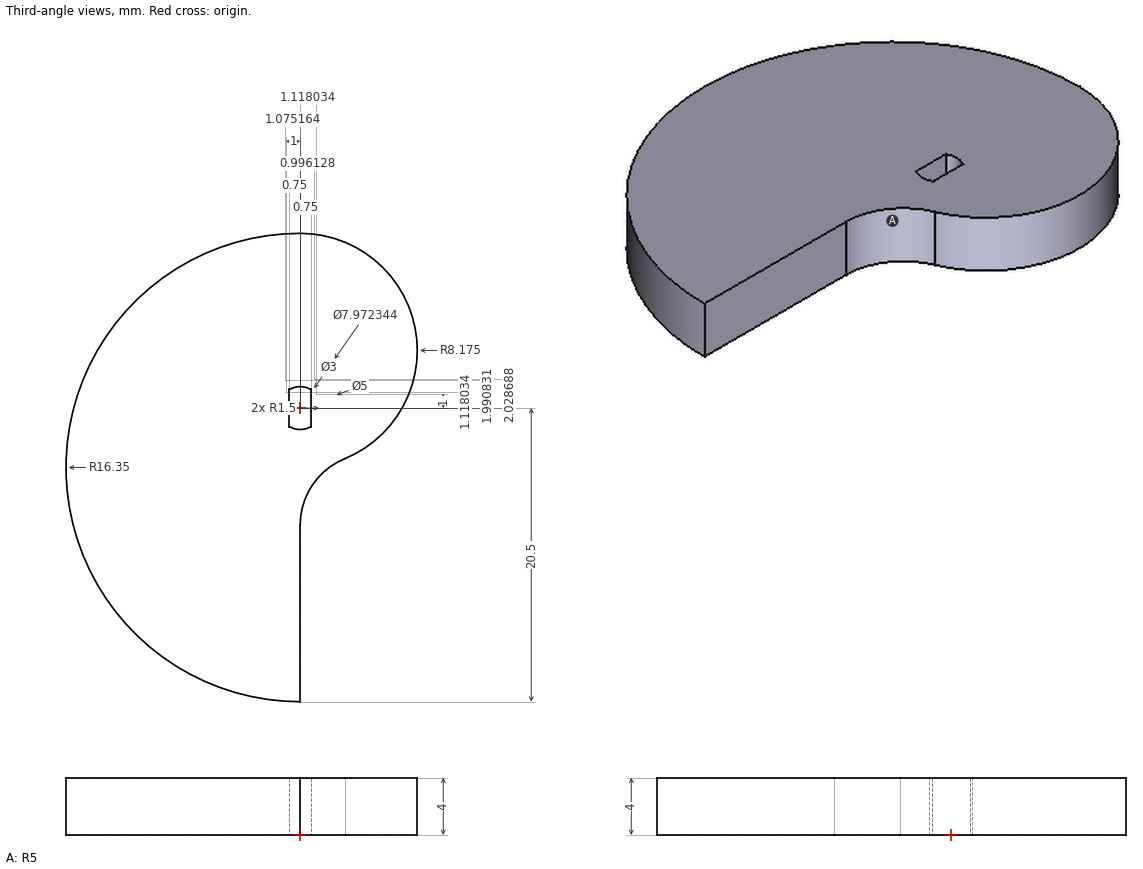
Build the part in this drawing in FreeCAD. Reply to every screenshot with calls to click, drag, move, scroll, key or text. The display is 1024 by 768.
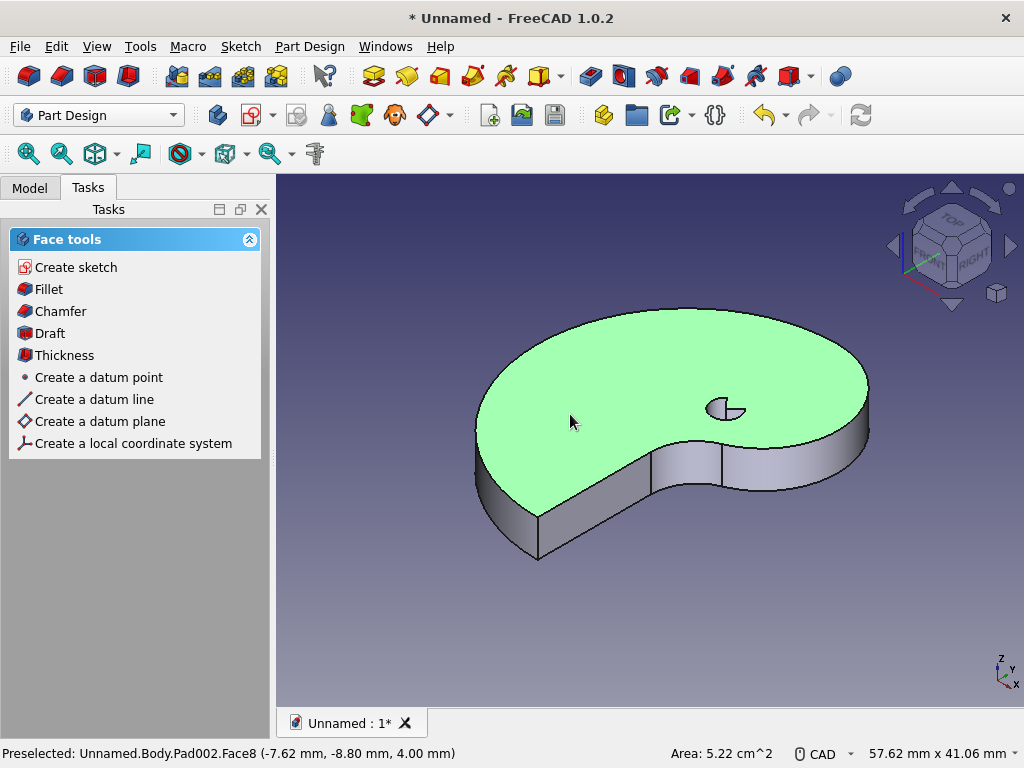
click(250, 116)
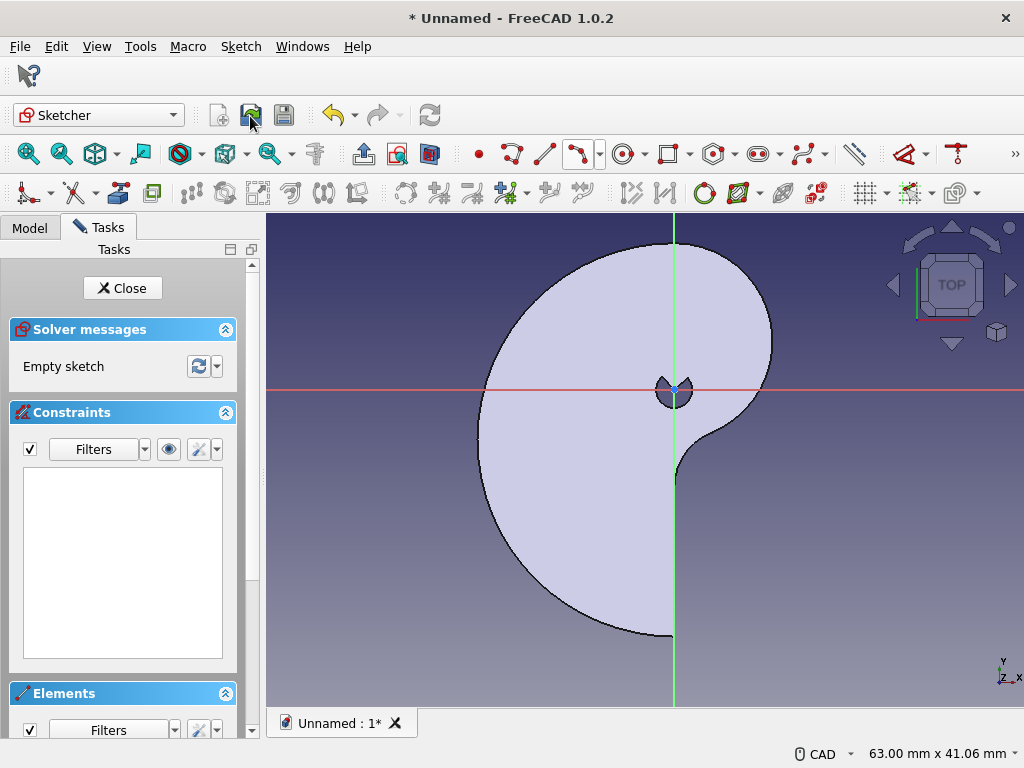
scroll(686, 381, up, 11)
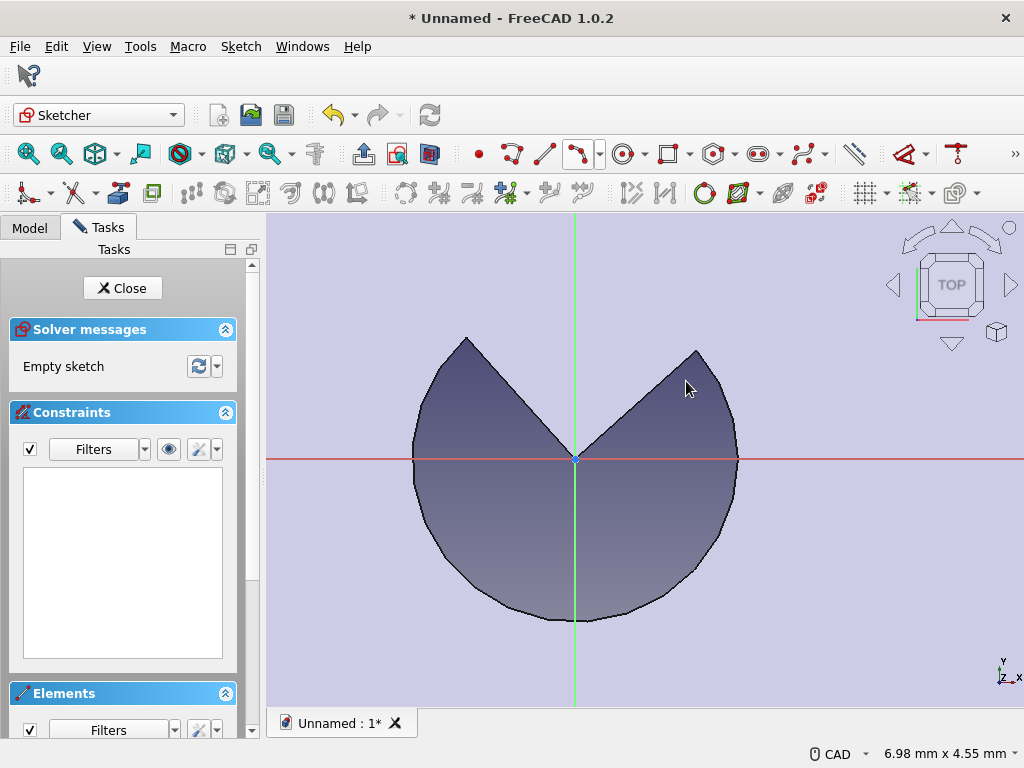
key(g)
key(c)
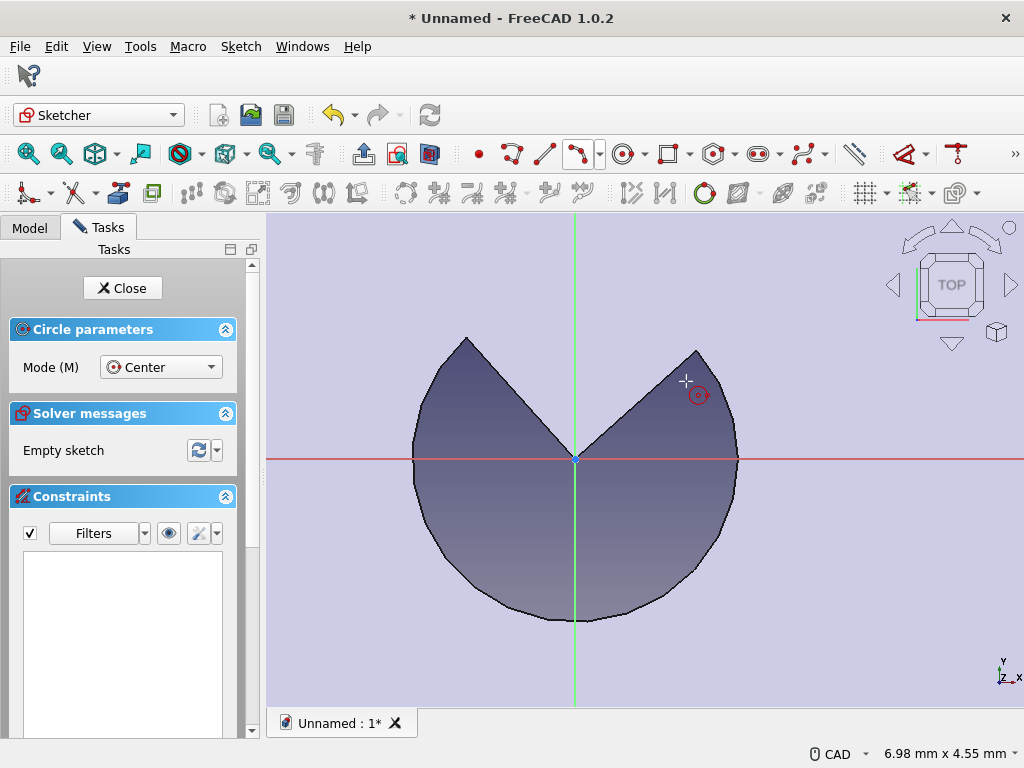
click(575, 459)
move(690, 344)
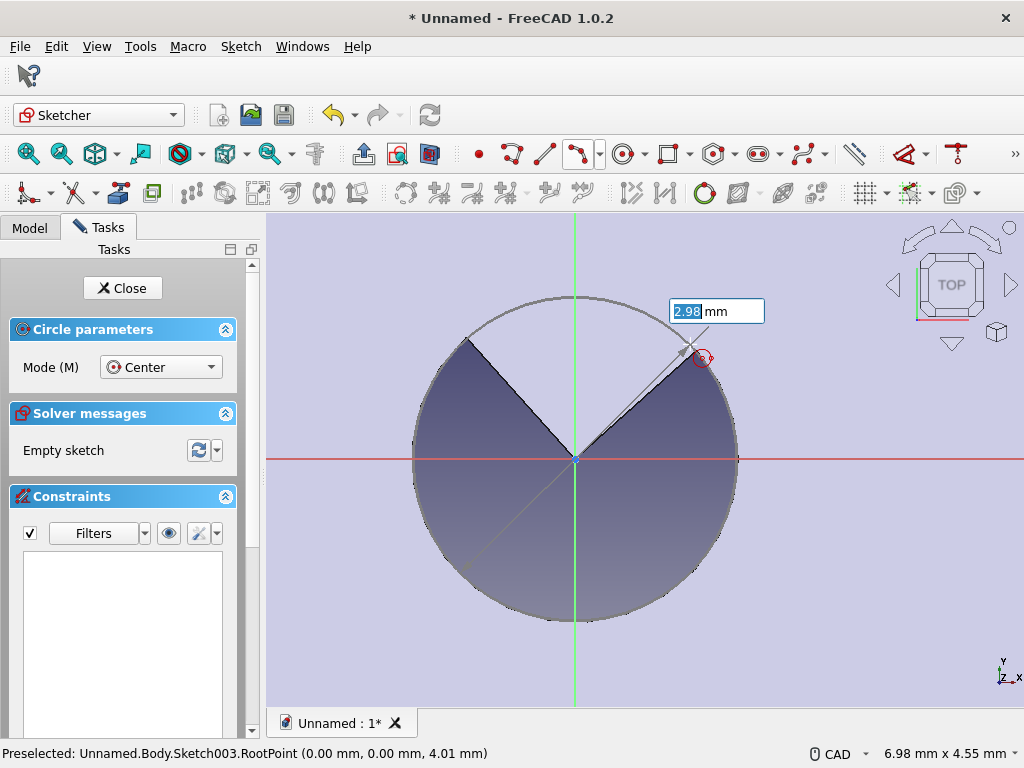
text(3)
key(Return)
key(Escape)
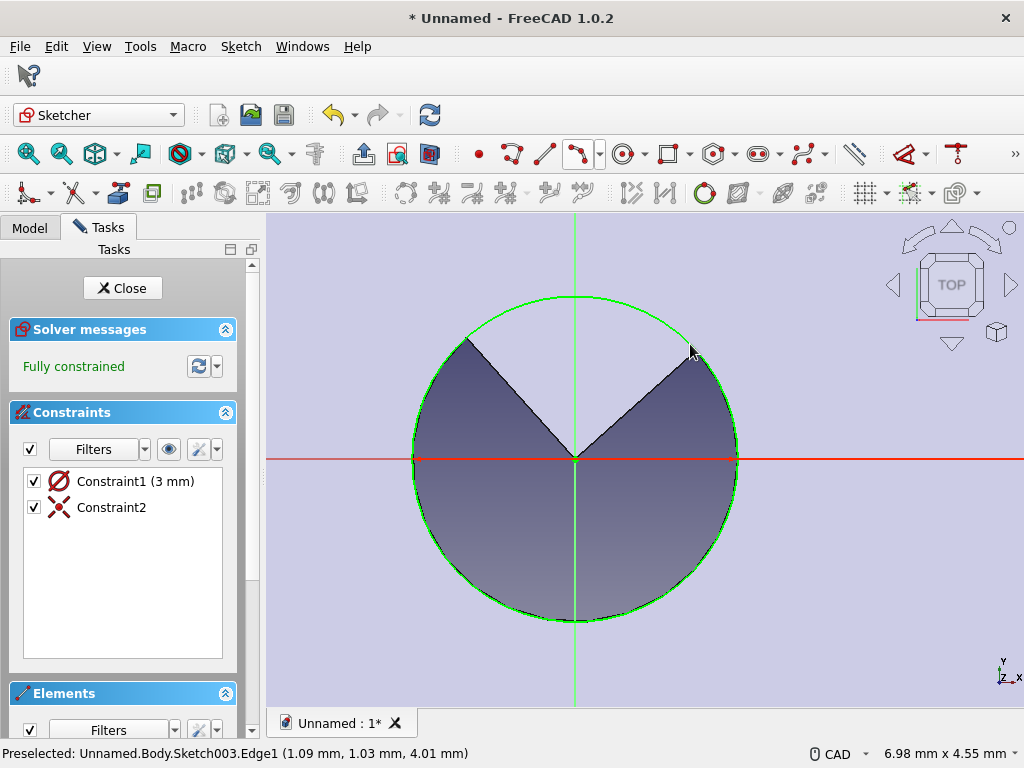
click(123, 288)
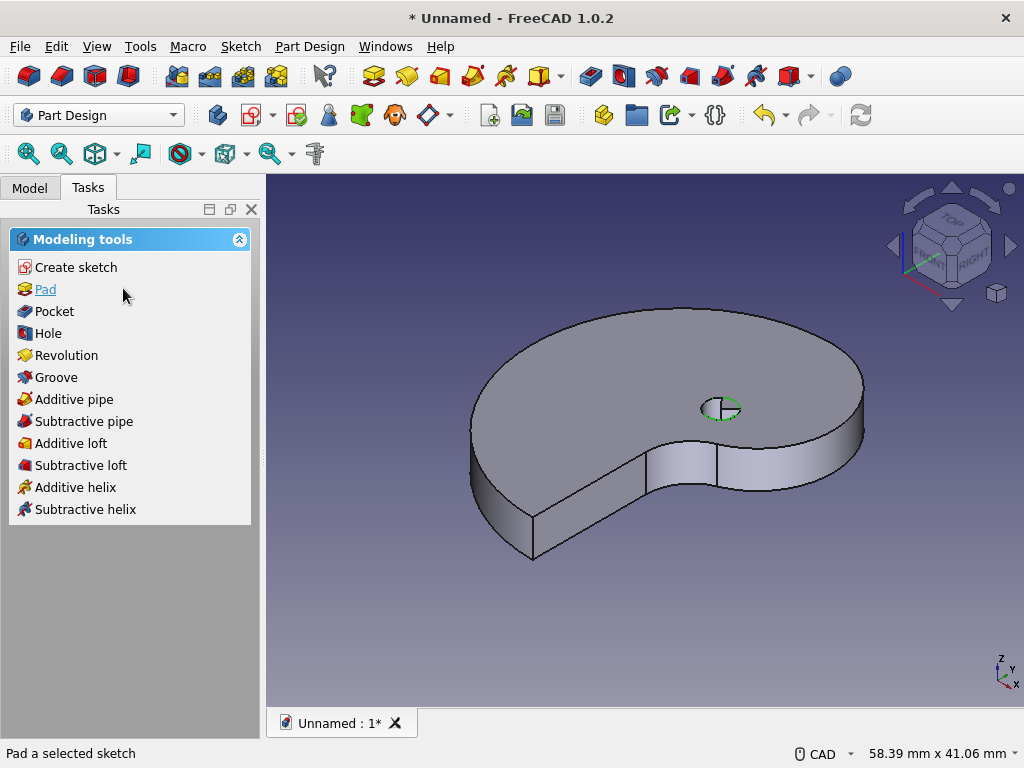
click(591, 76)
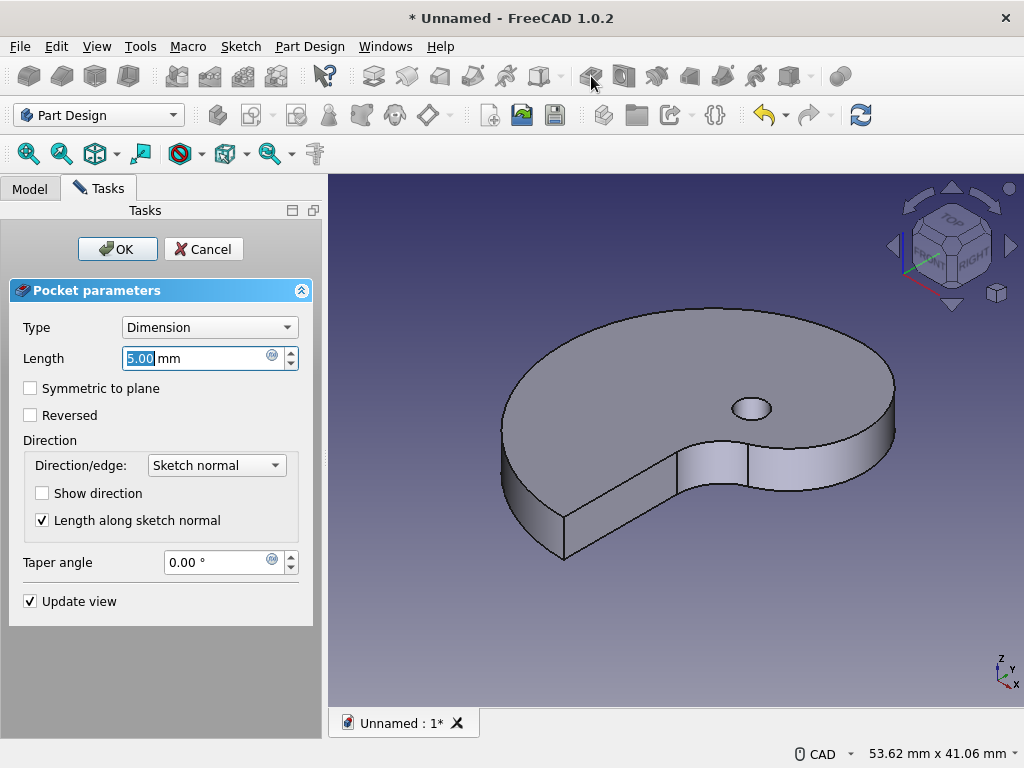
click(210, 328)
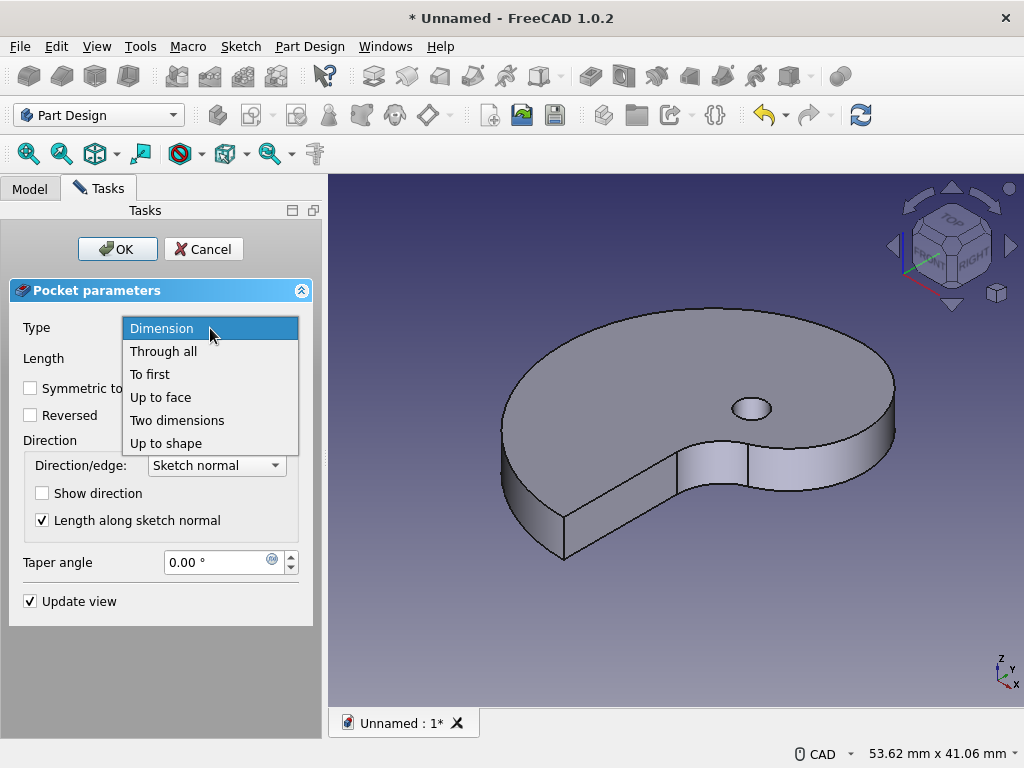
click(208, 352)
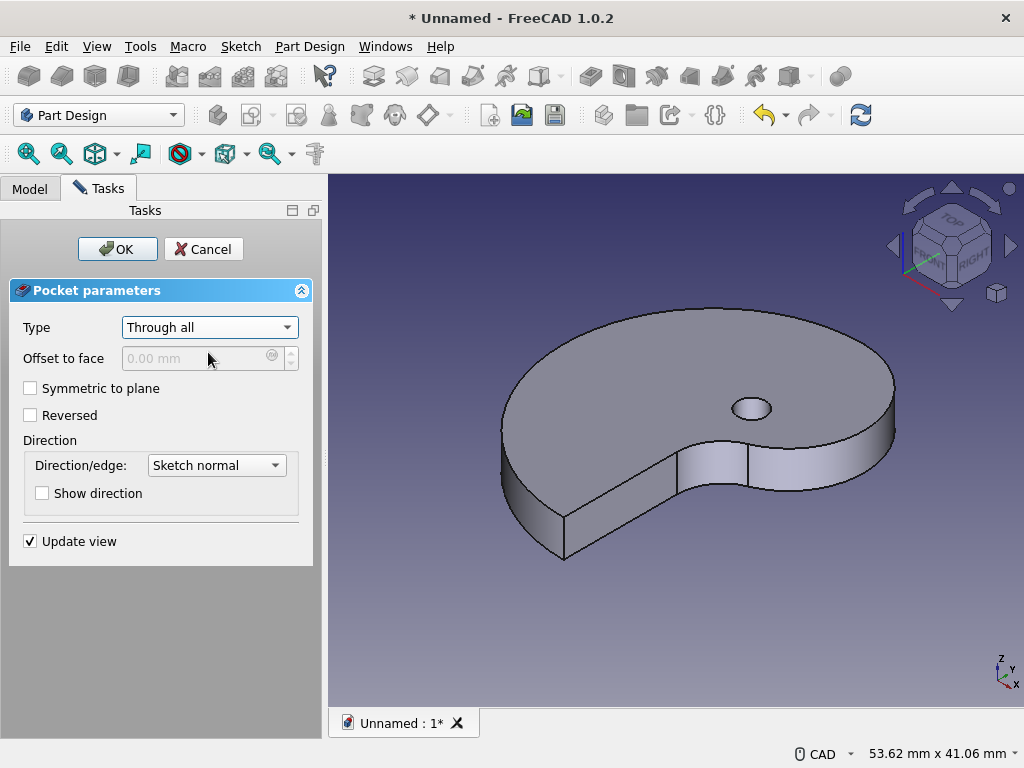
click(118, 249)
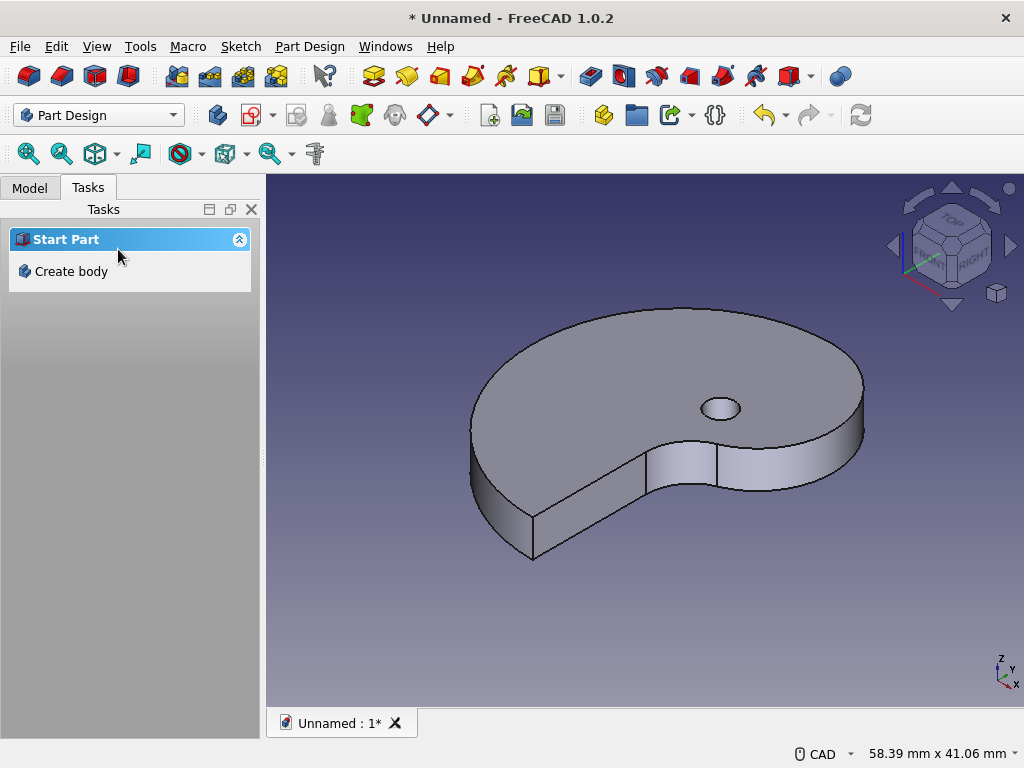
click(570, 414)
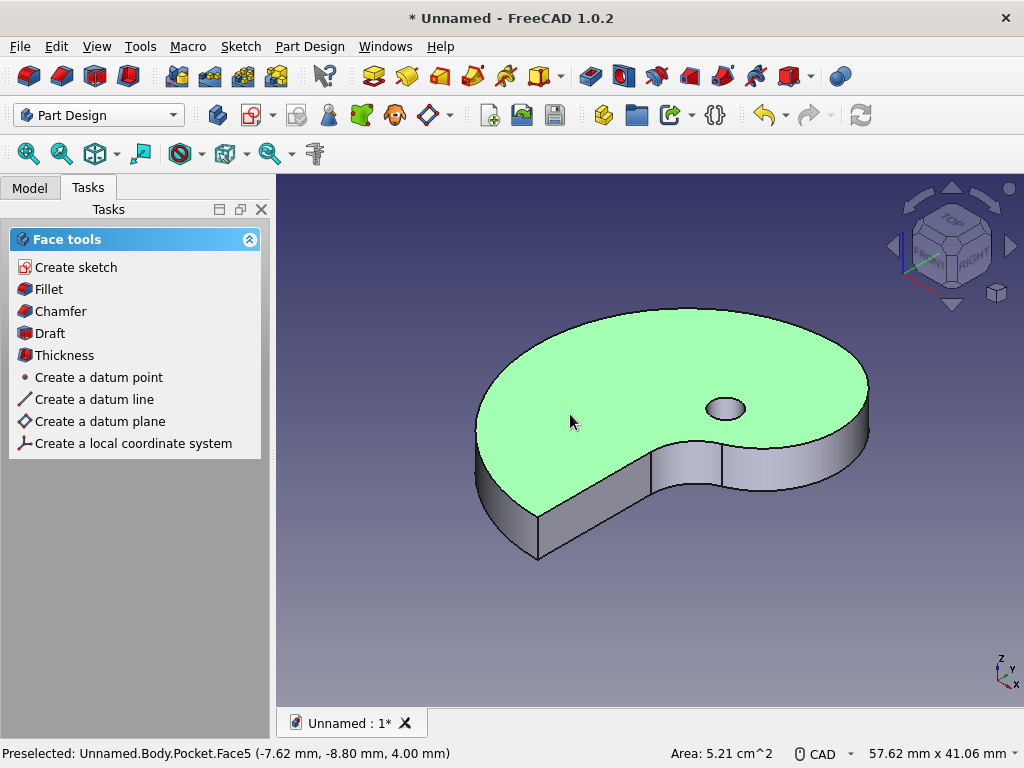
click(250, 116)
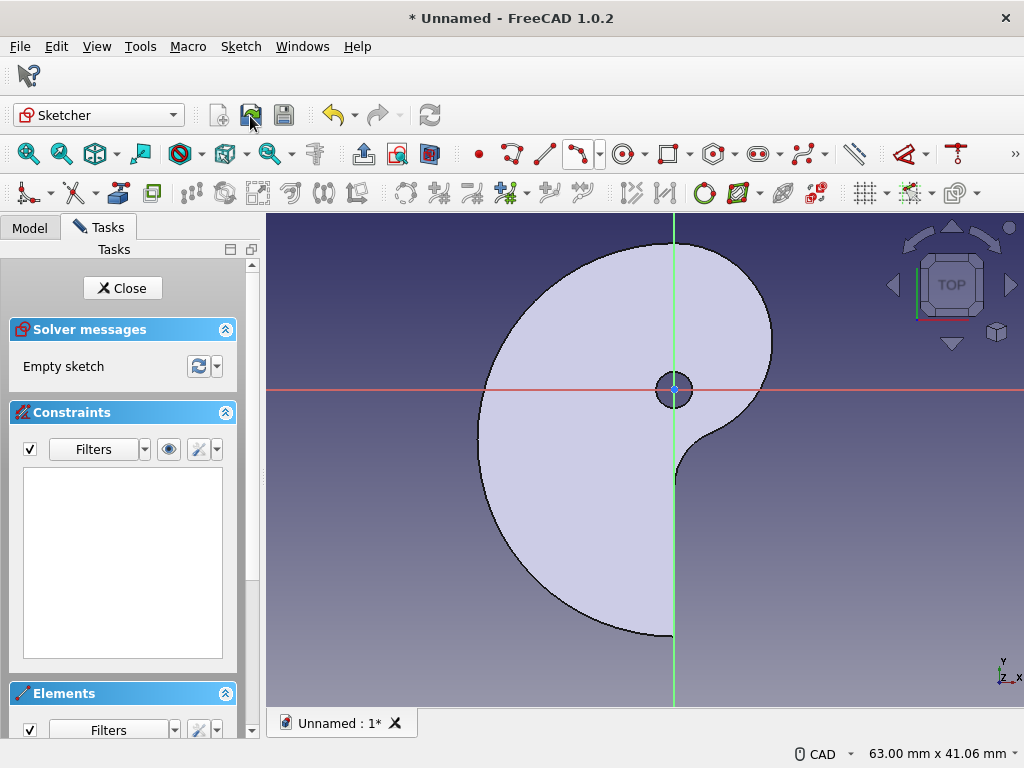
scroll(686, 381, up, 11)